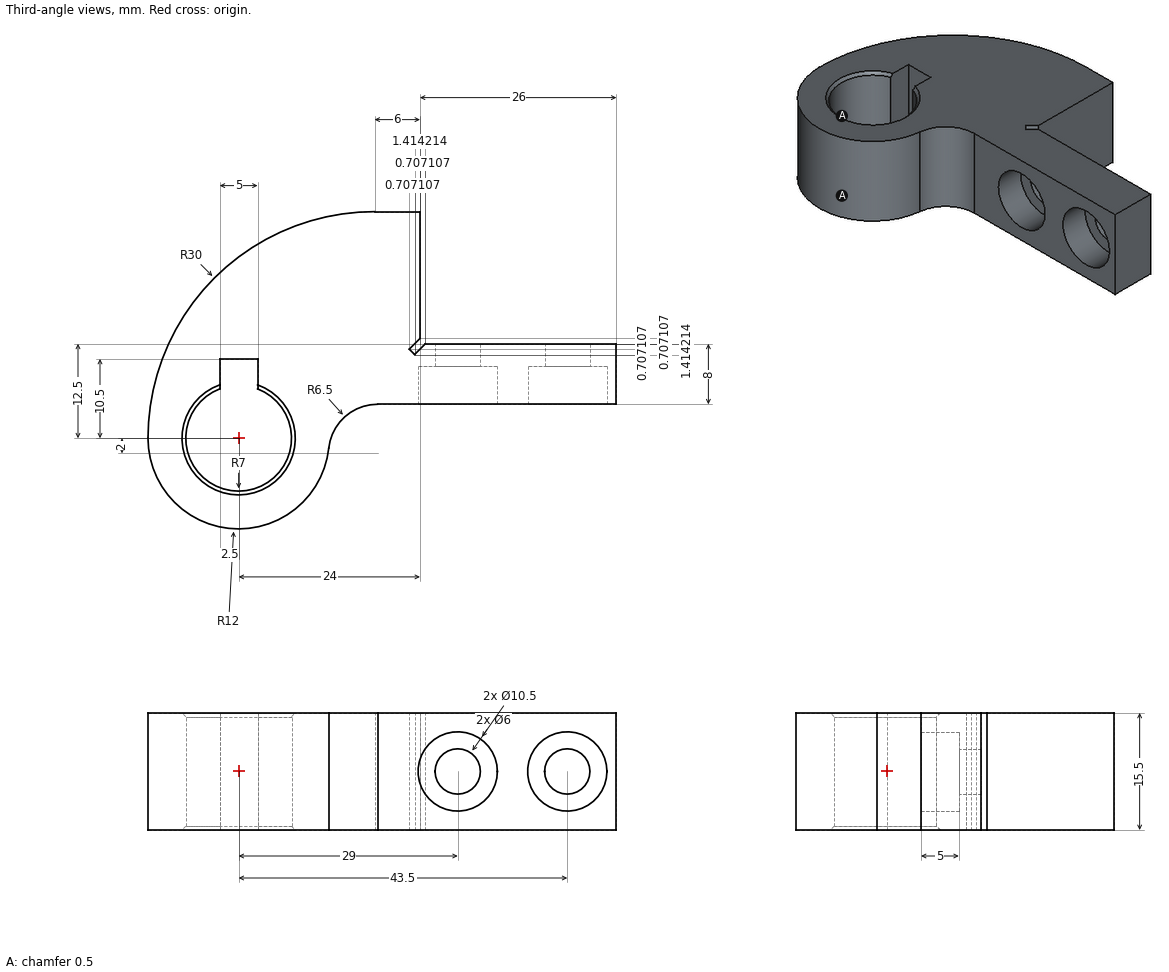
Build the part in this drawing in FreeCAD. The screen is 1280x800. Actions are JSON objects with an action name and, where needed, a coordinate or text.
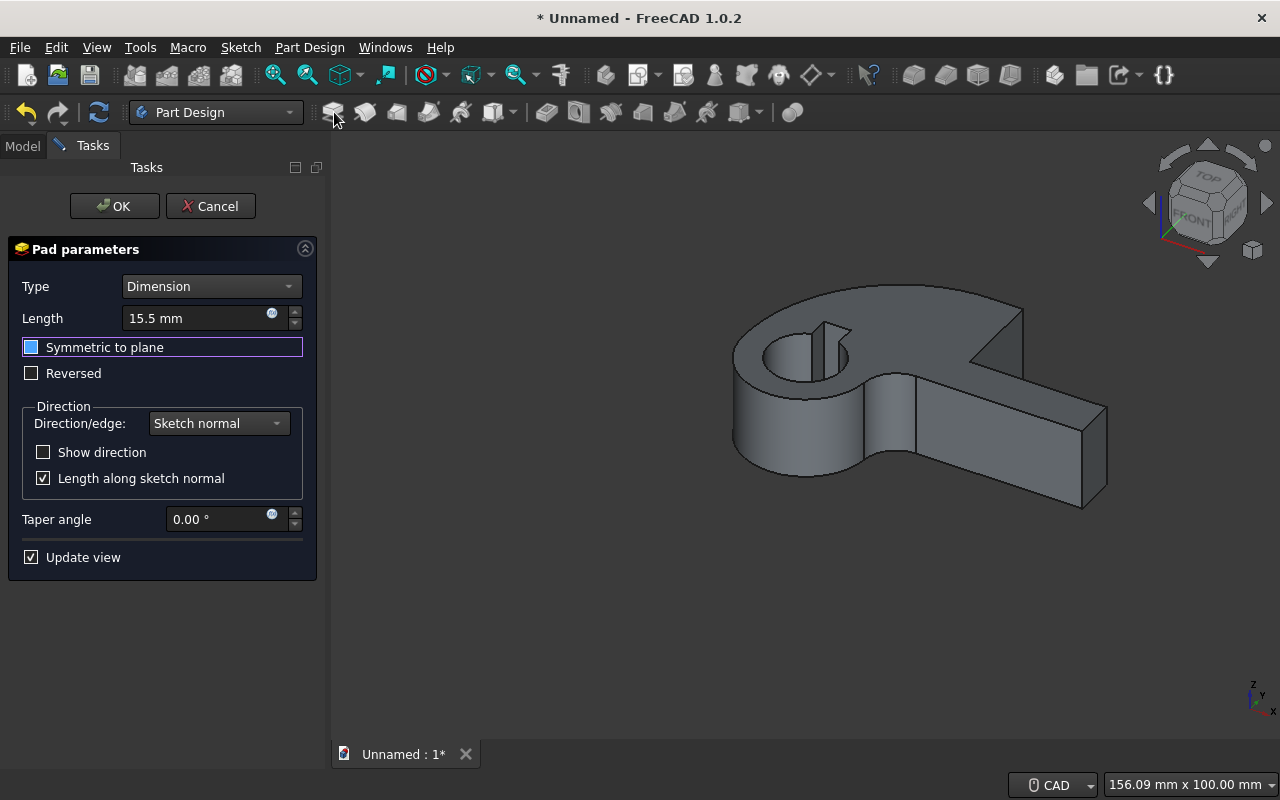
{"action": "left_click", "coordinate": [30, 347]}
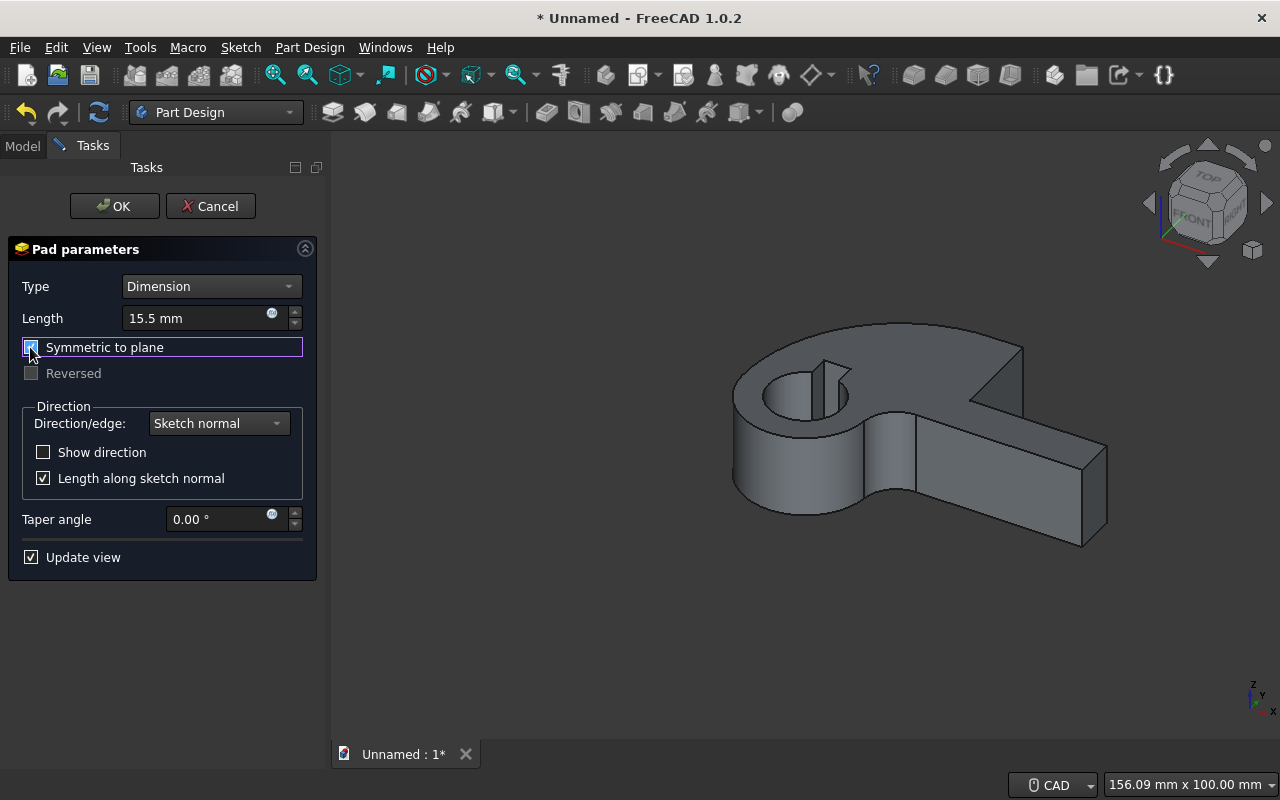
{"action": "left_click", "coordinate": [115, 206]}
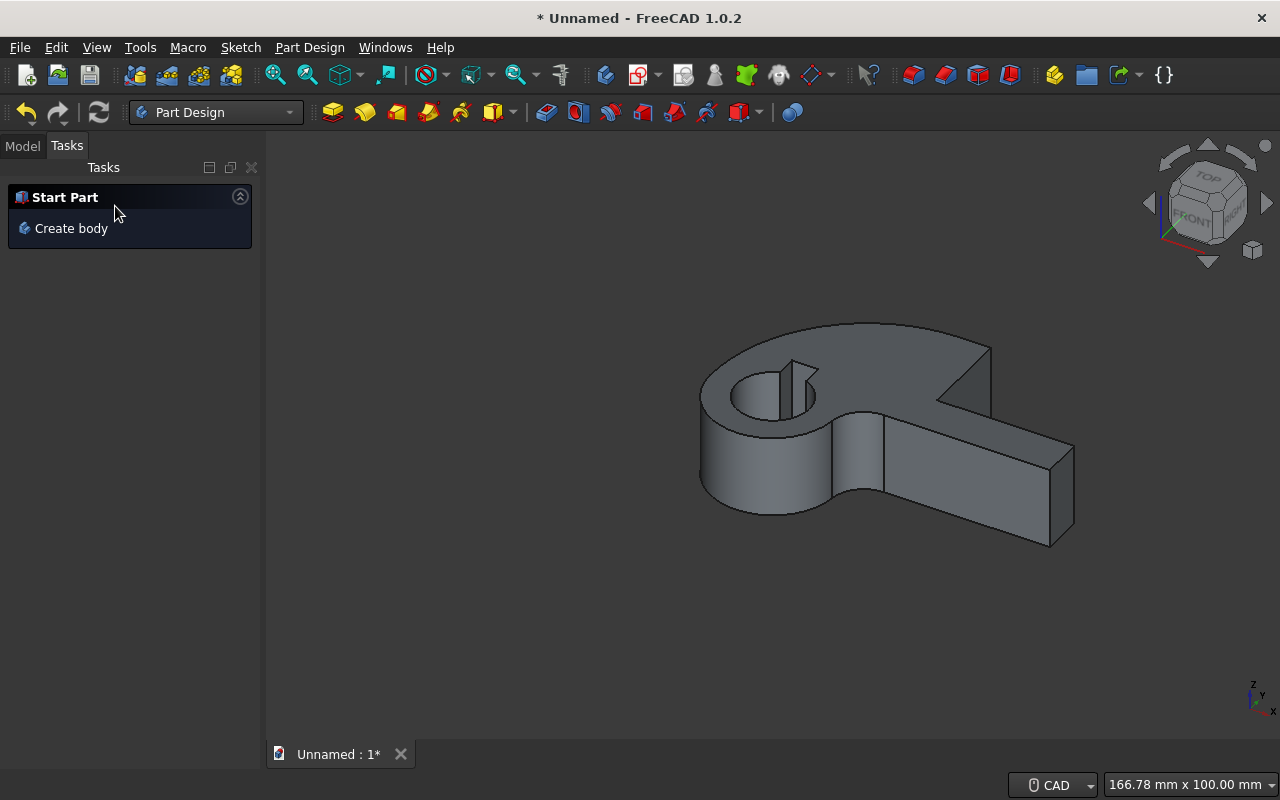
{"action": "key", "text": "4"}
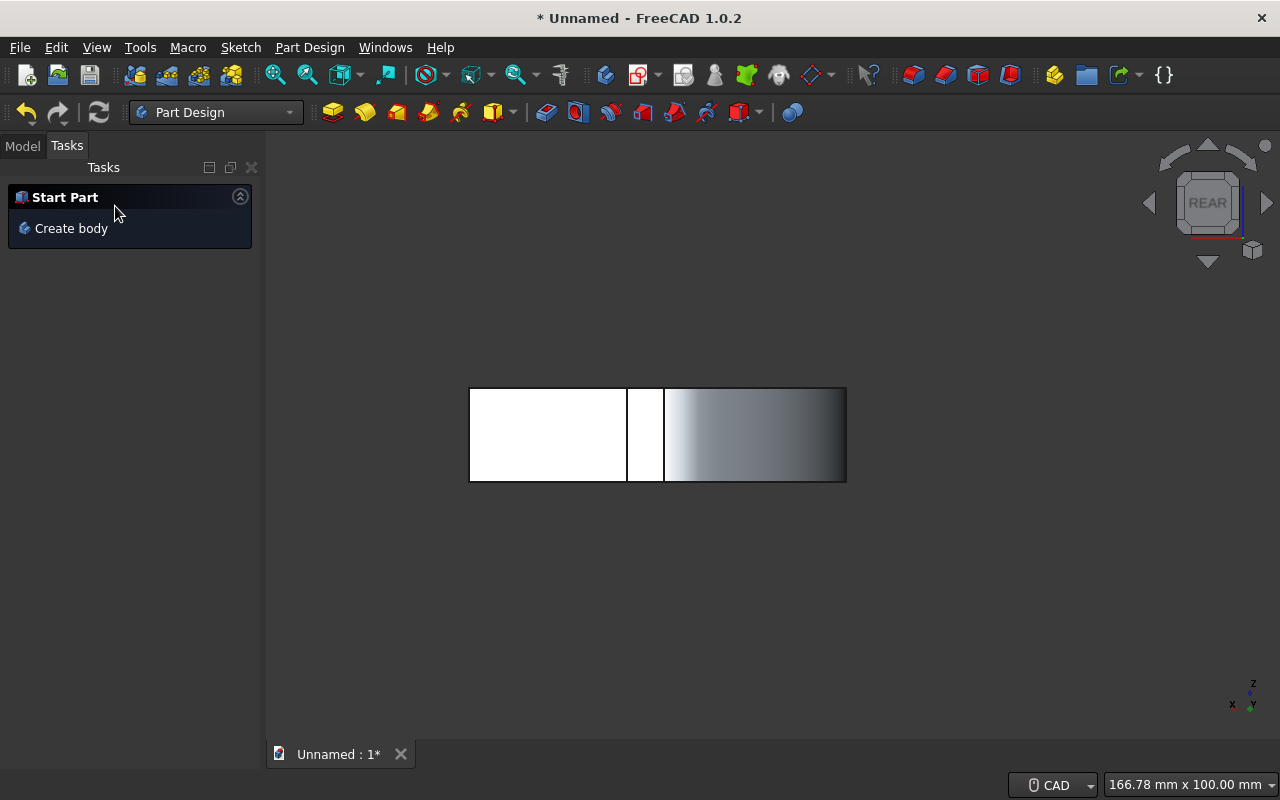
{"action": "left_click", "coordinate": [276, 76]}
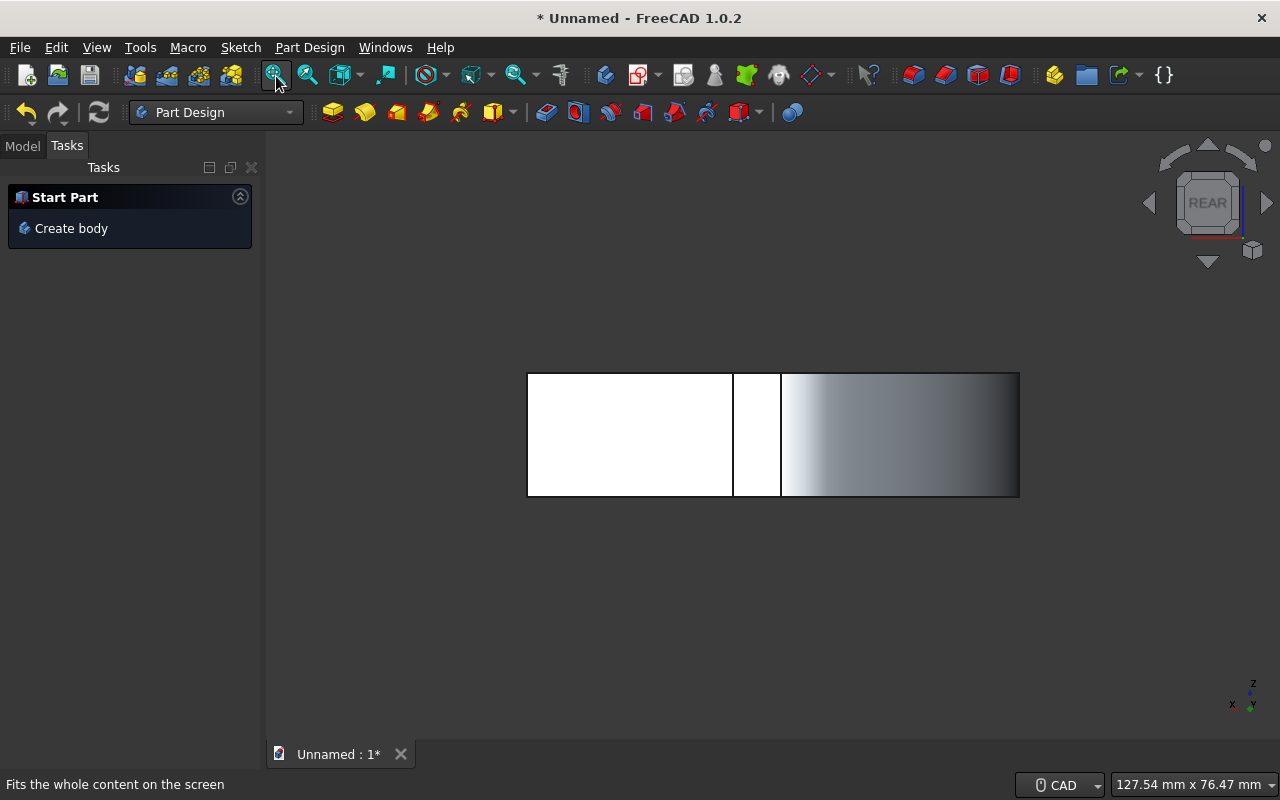
{"action": "left_click", "coordinate": [600, 434]}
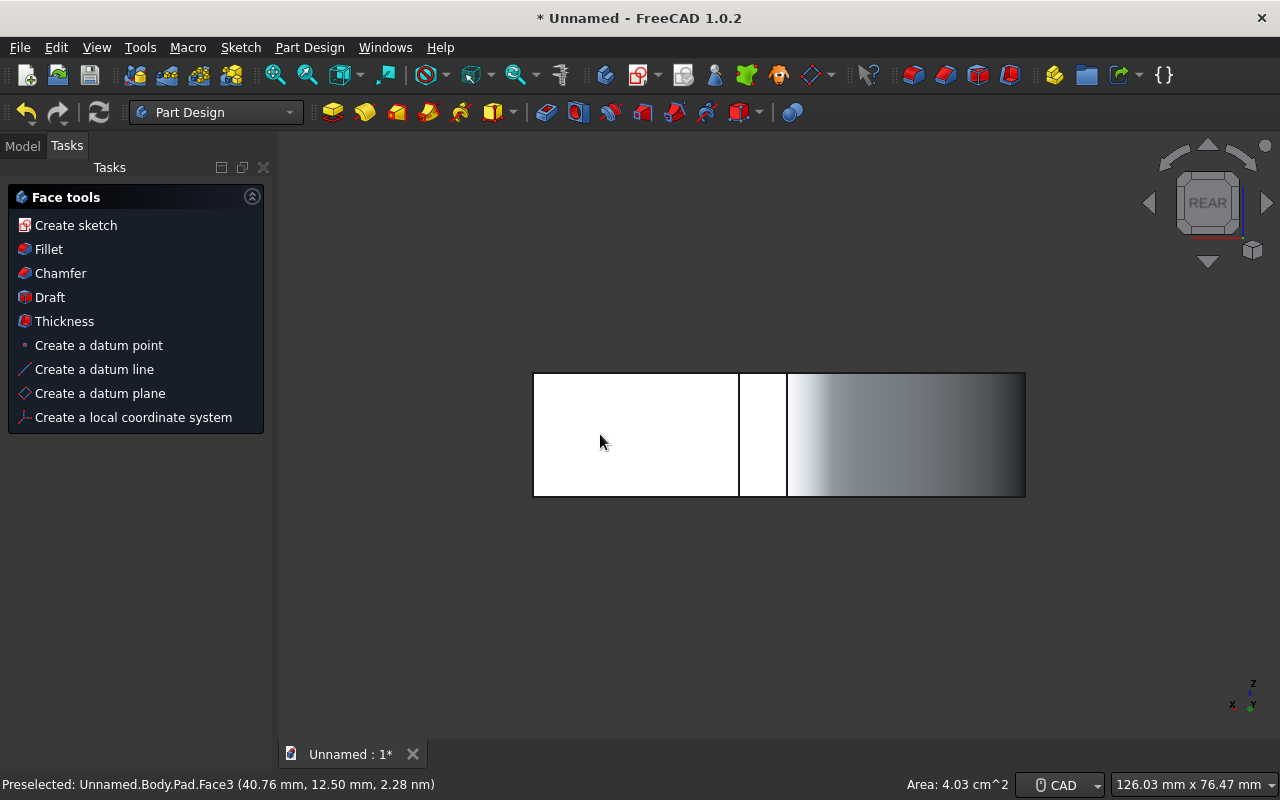
{"action": "left_click", "coordinate": [638, 76]}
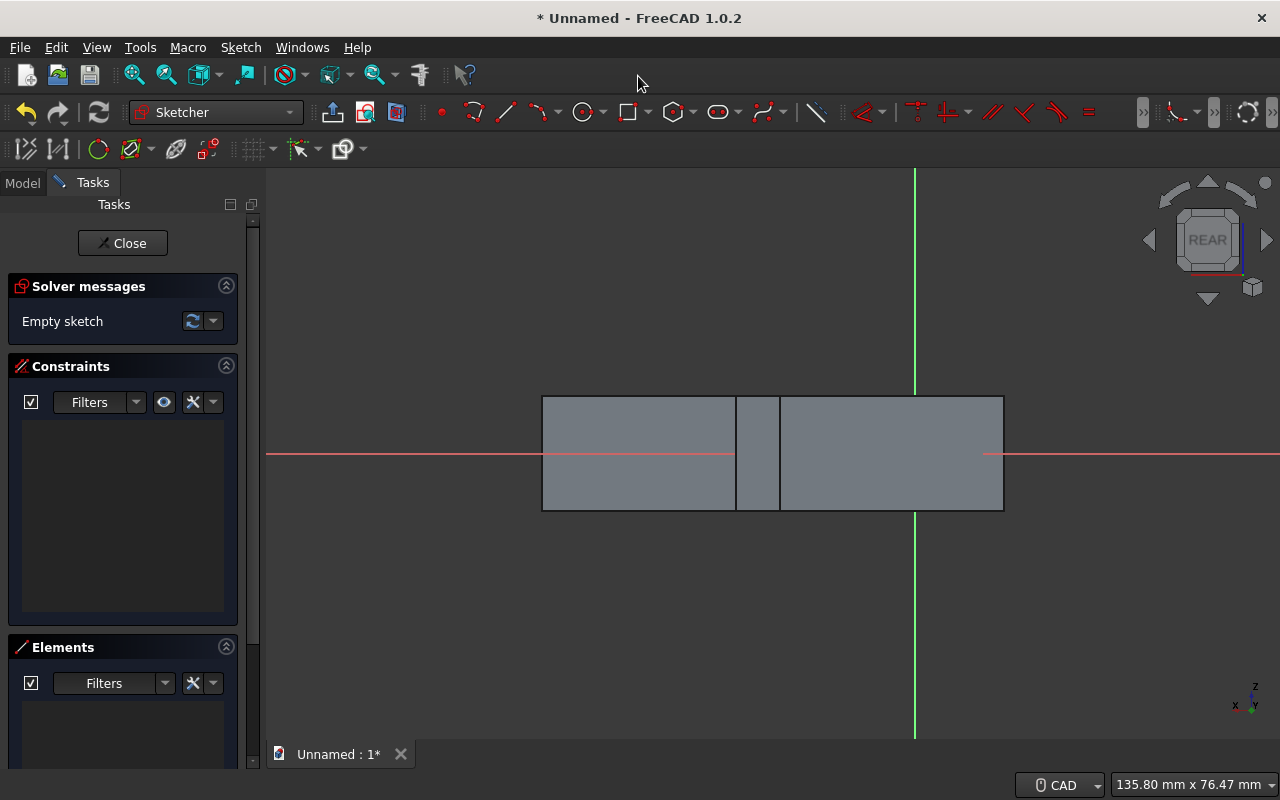
{"action": "left_click", "coordinate": [398, 112]}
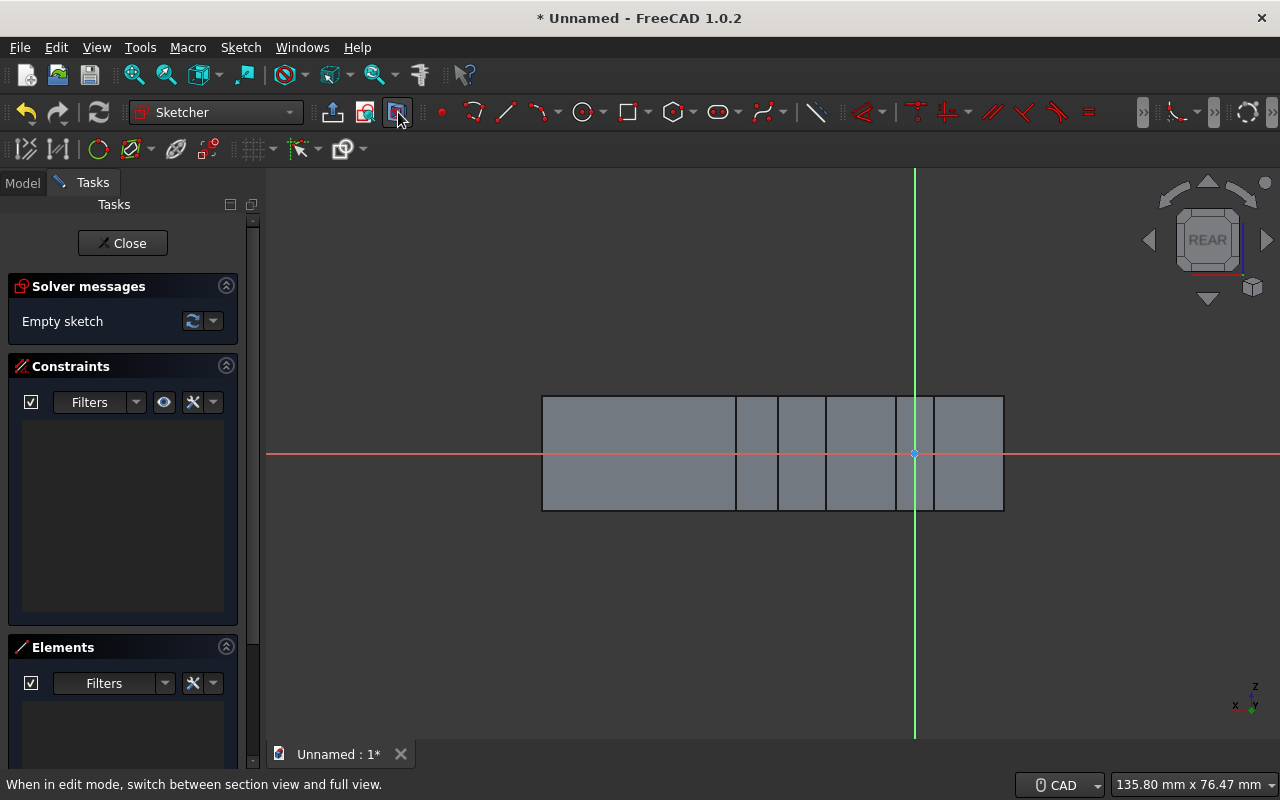
{"action": "scroll", "coordinate": [786, 453], "scroll_direction": "up", "scroll_amount": 3}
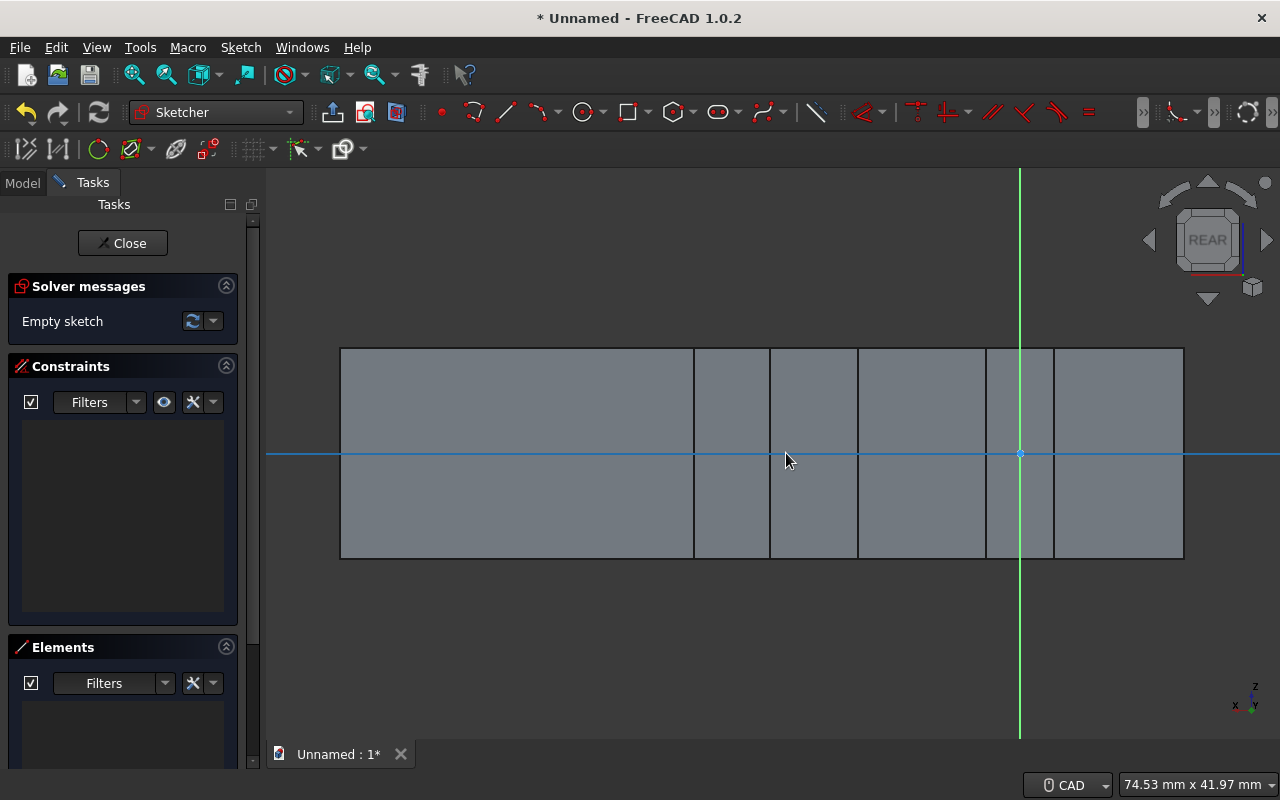
{"action": "left_click", "coordinate": [584, 112]}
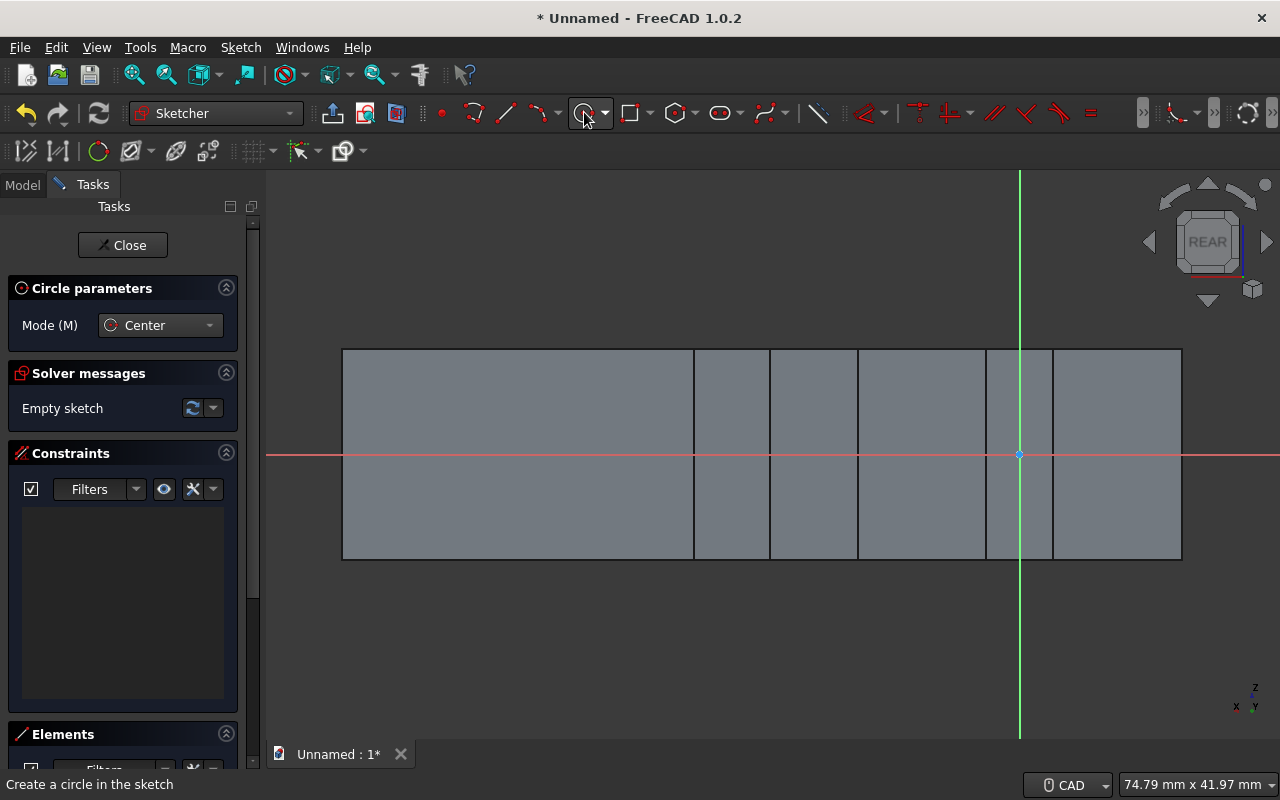
{"action": "left_click", "coordinate": [626, 454]}
{"action": "left_click", "coordinate": [655, 426]}